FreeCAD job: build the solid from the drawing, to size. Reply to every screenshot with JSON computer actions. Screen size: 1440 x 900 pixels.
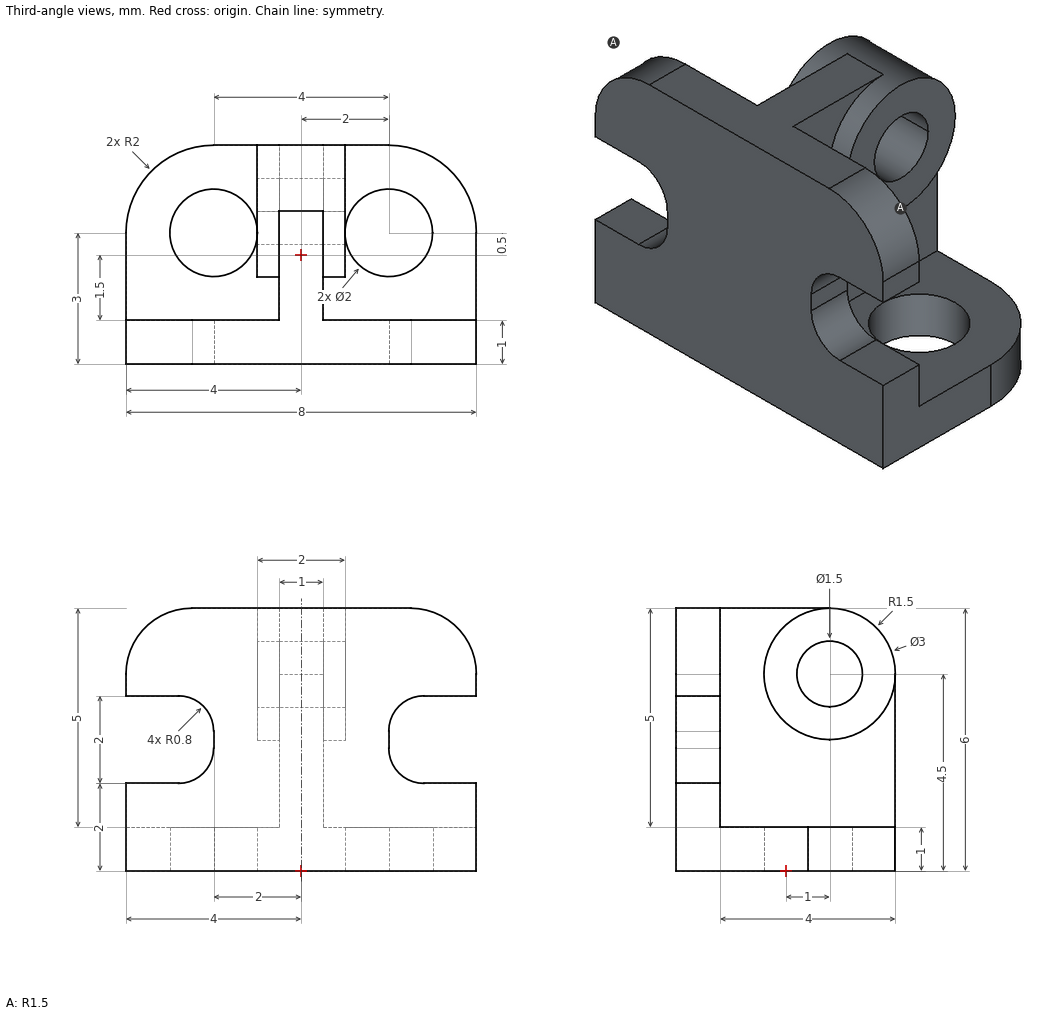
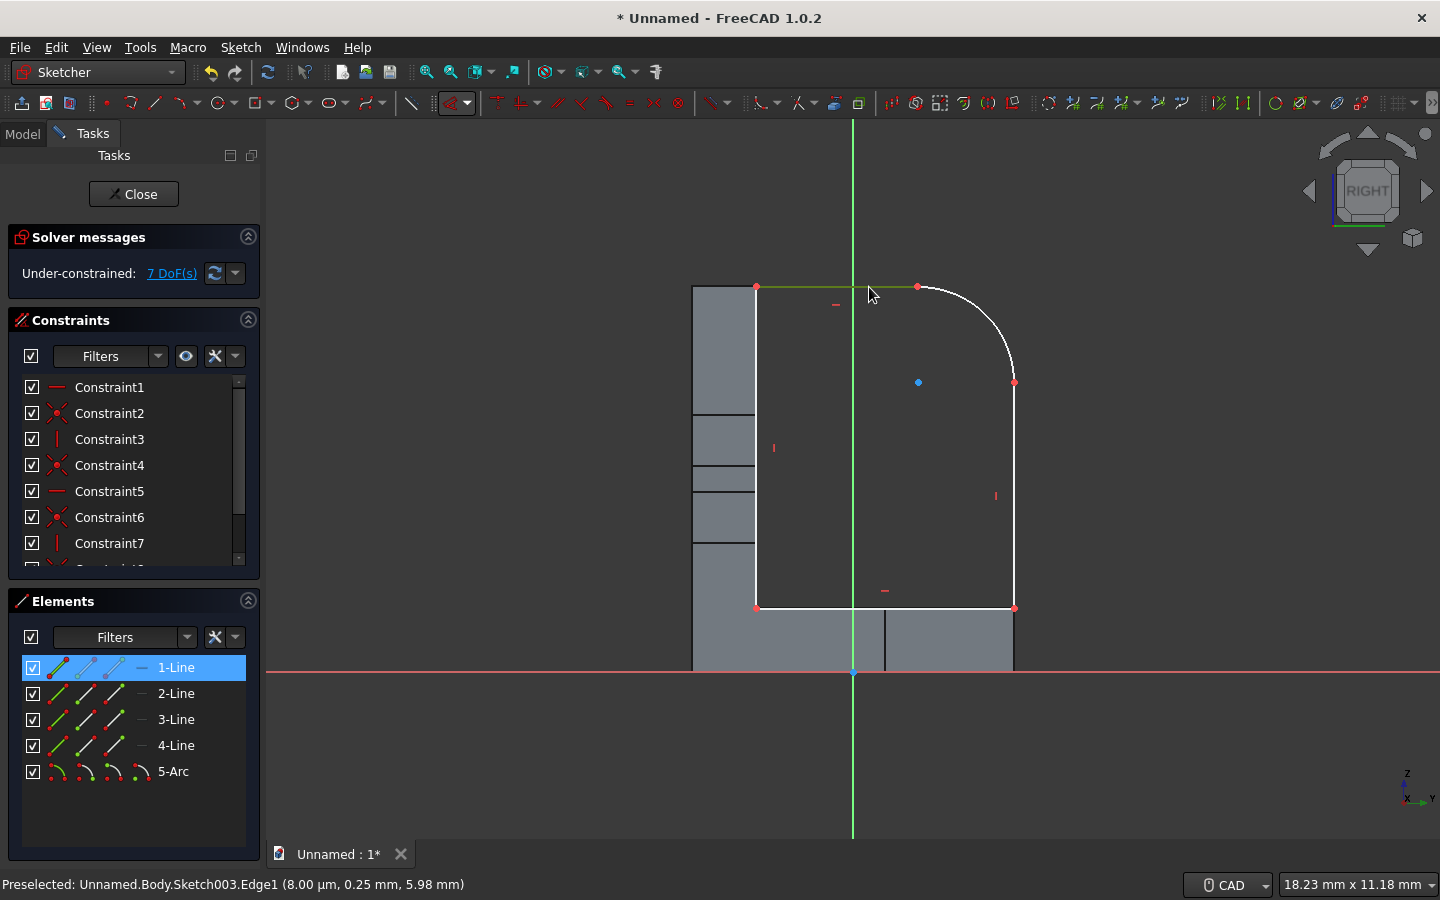
{"action": "left_click", "coordinate": [1004, 339]}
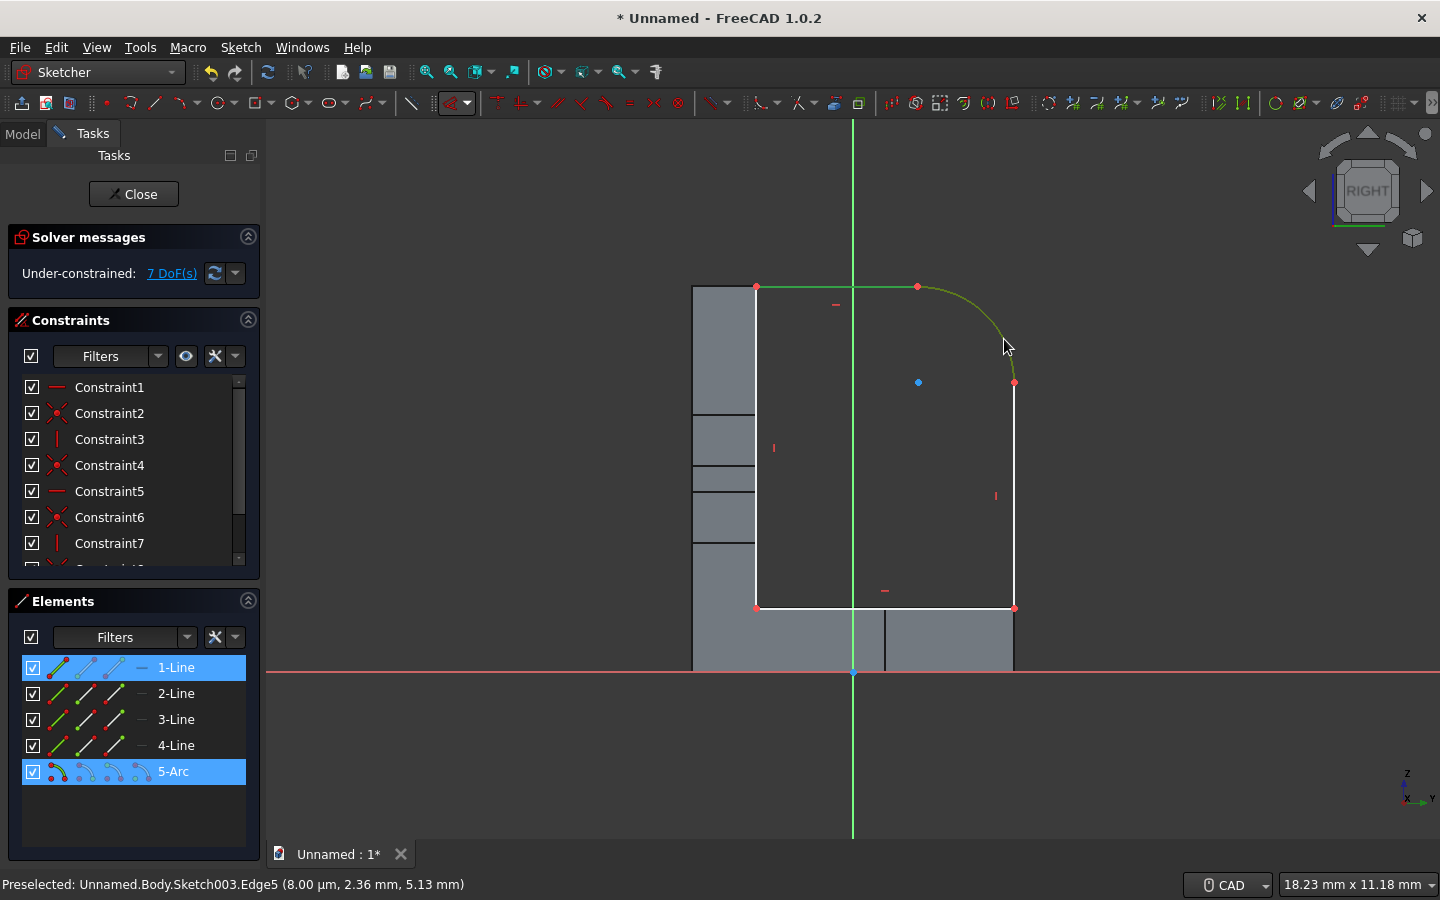
{"action": "left_click", "coordinate": [606, 104]}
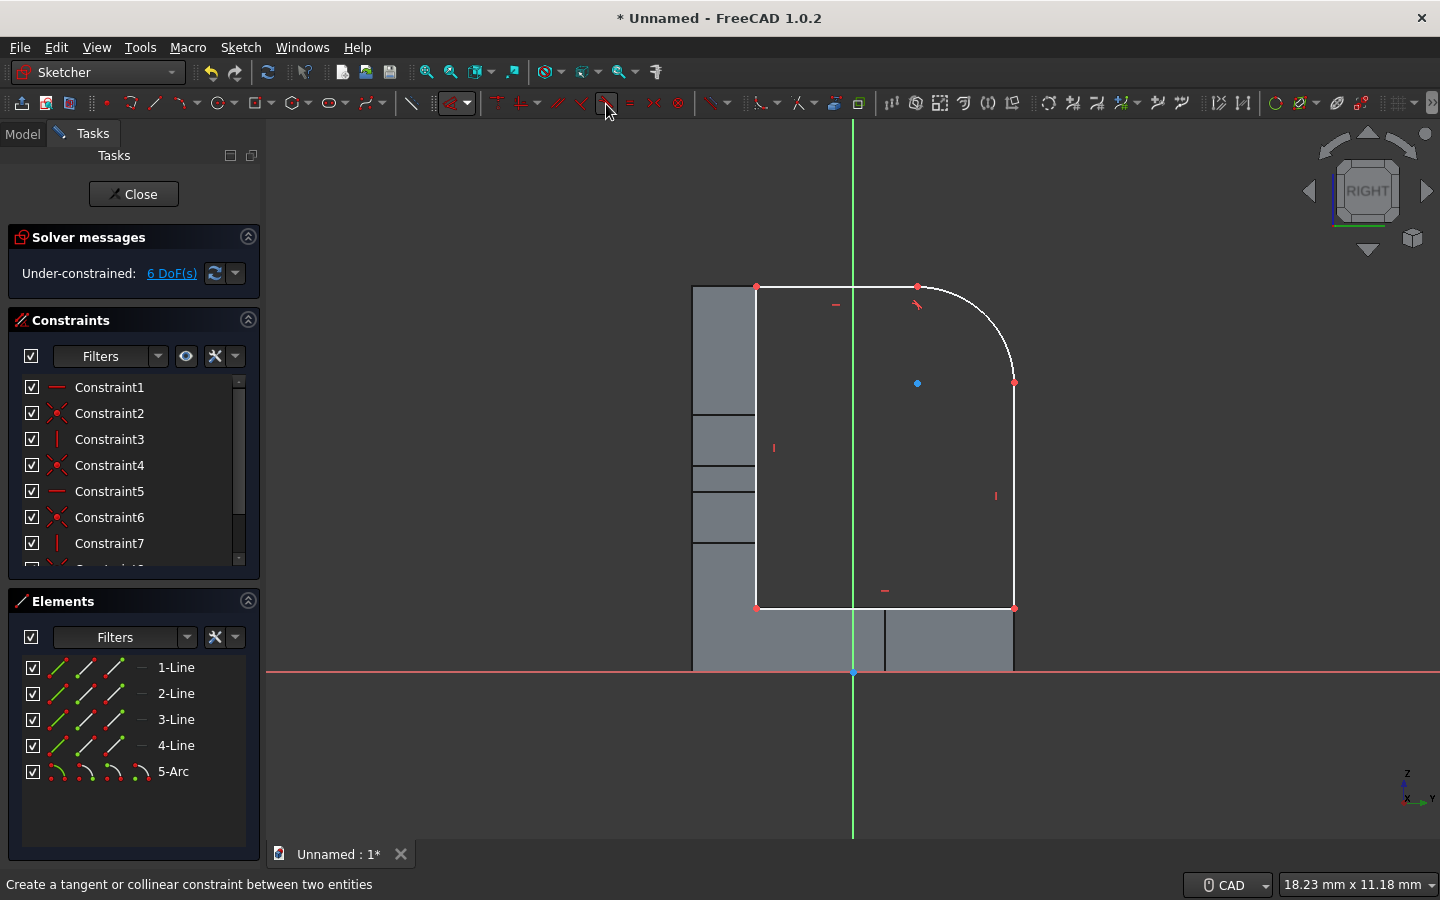
{"action": "left_click", "coordinate": [1014, 541]}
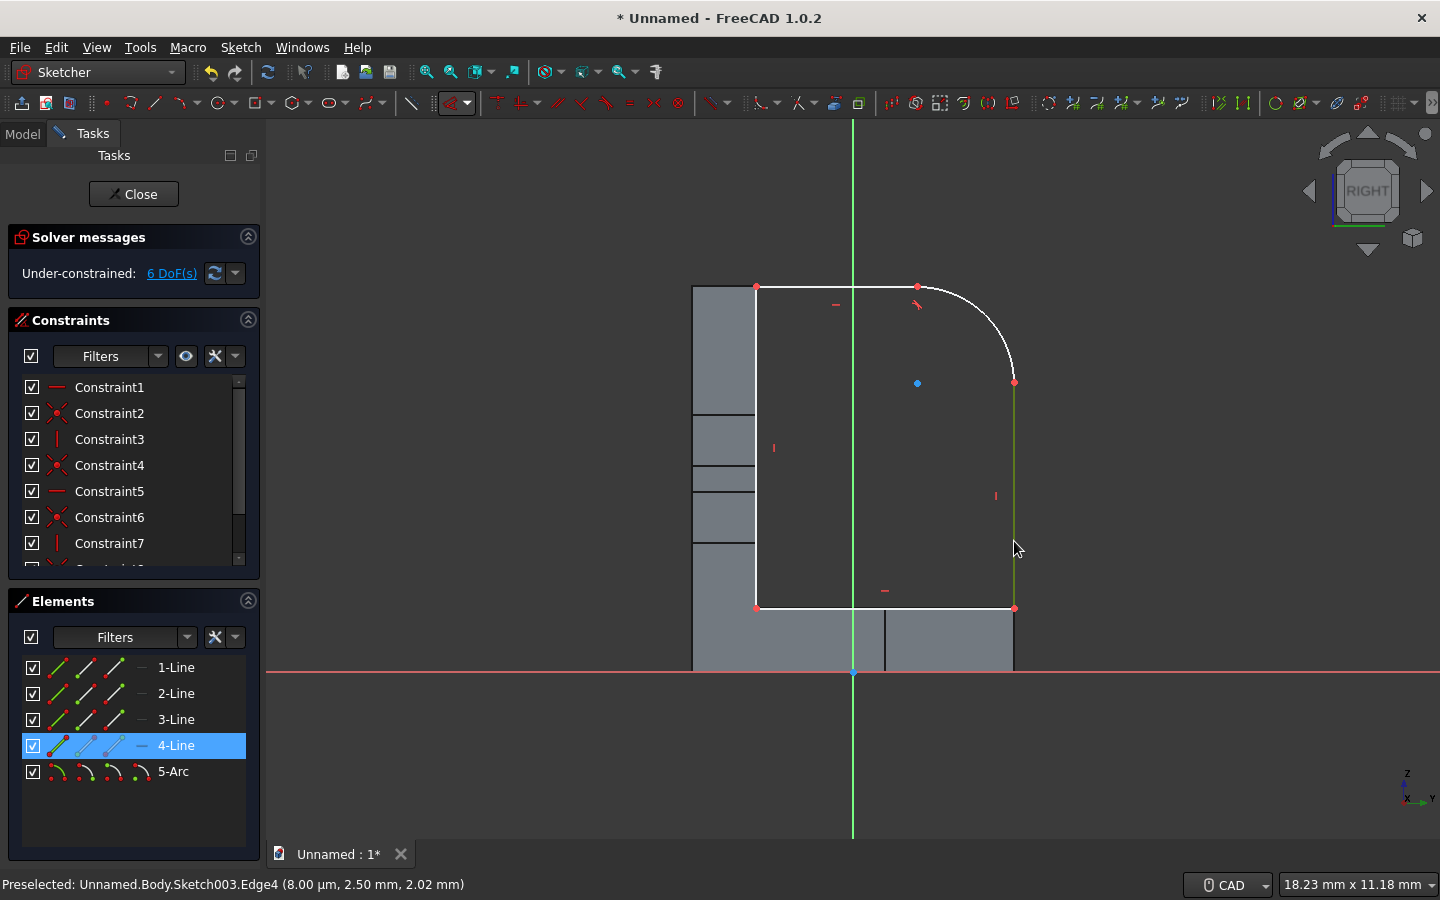
{"action": "left_click", "coordinate": [1003, 339]}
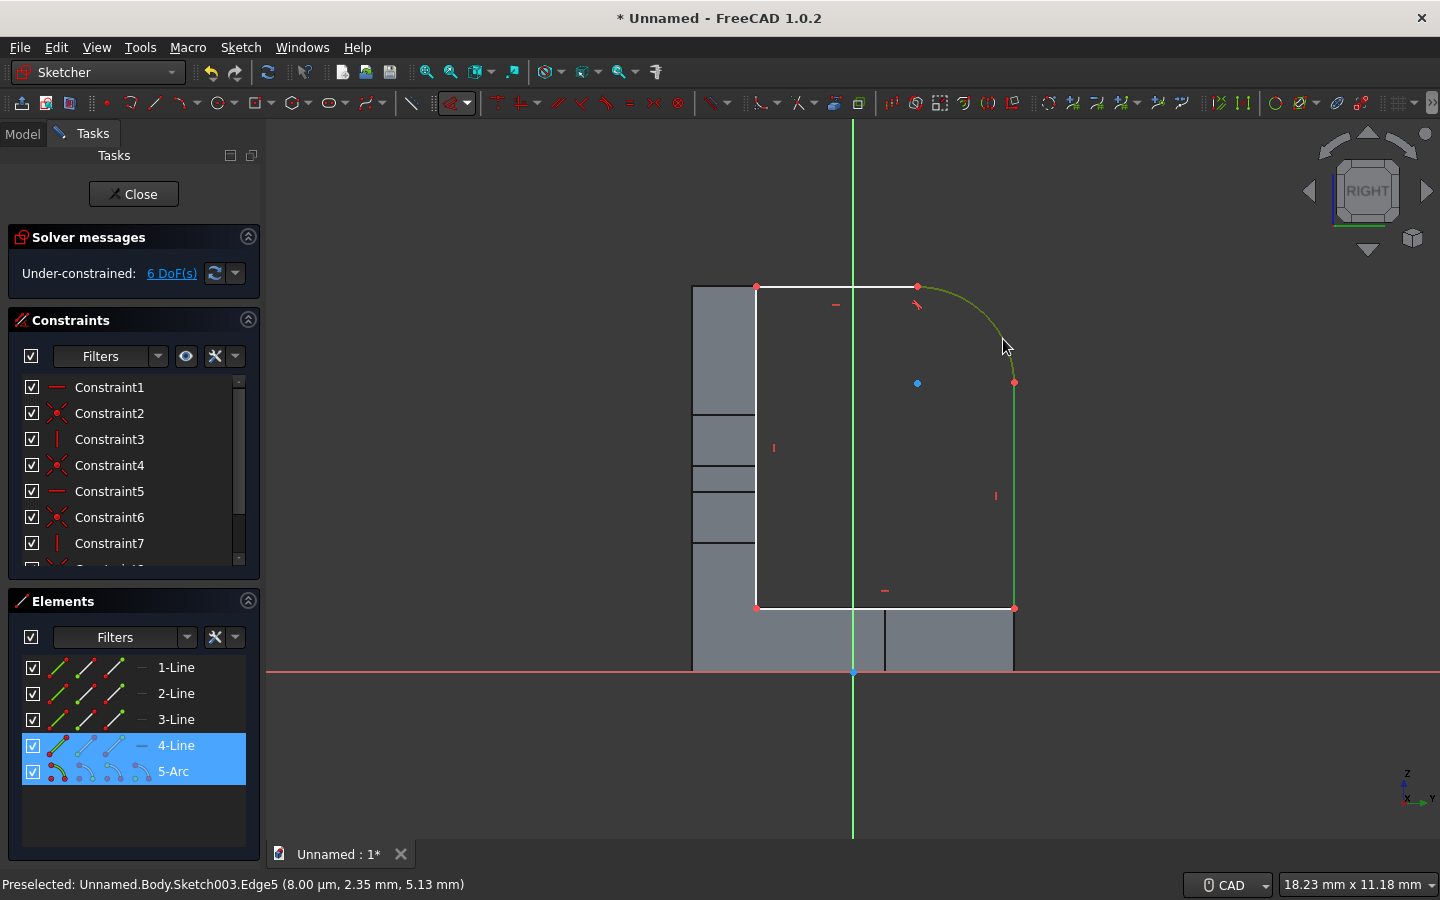
{"action": "left_click", "coordinate": [606, 104]}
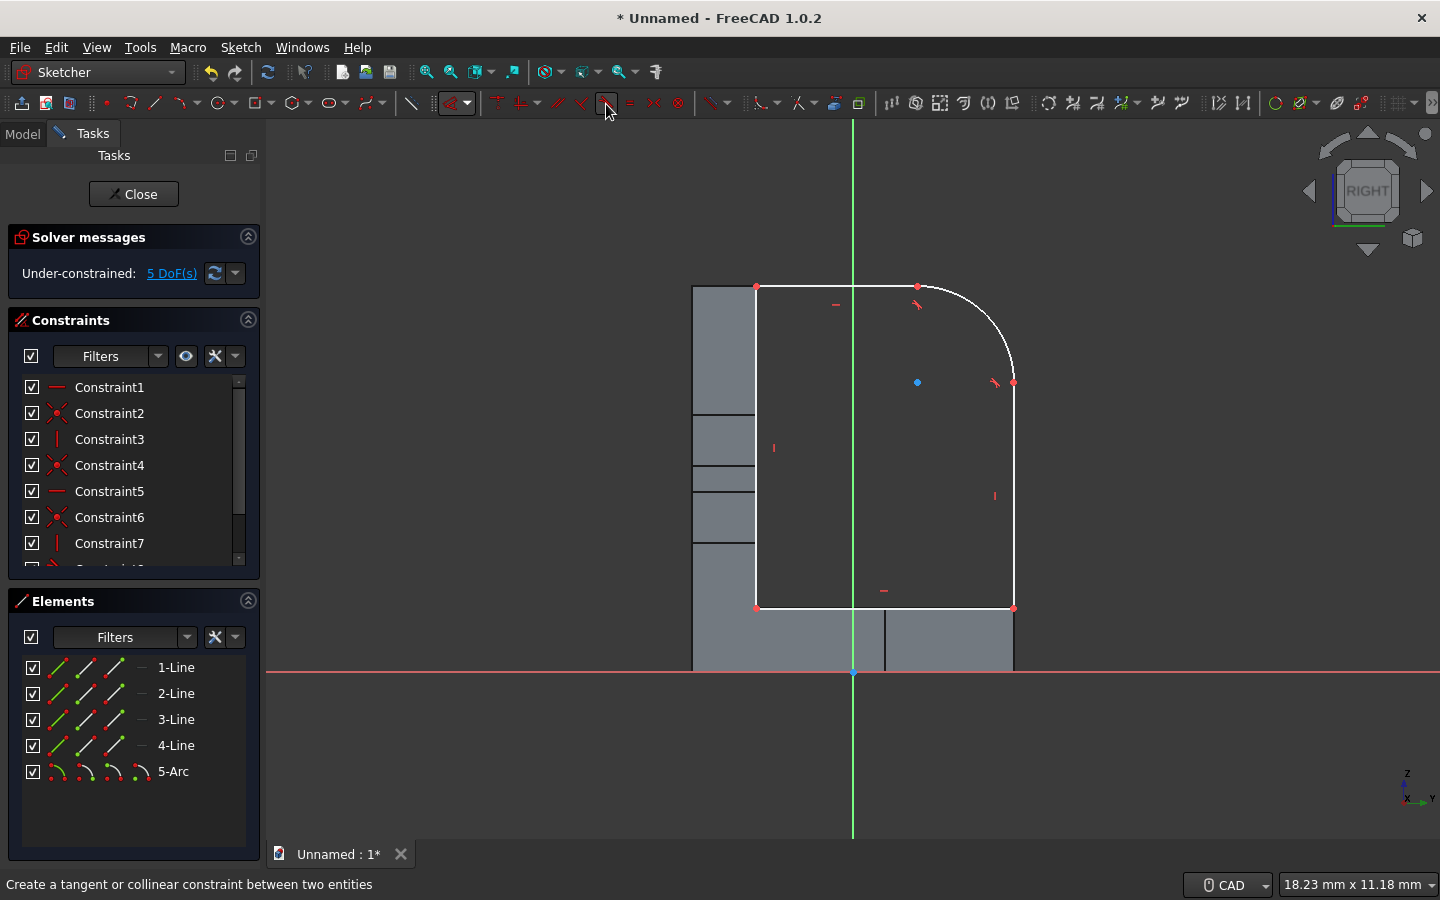
{"action": "left_click", "coordinate": [1003, 339]}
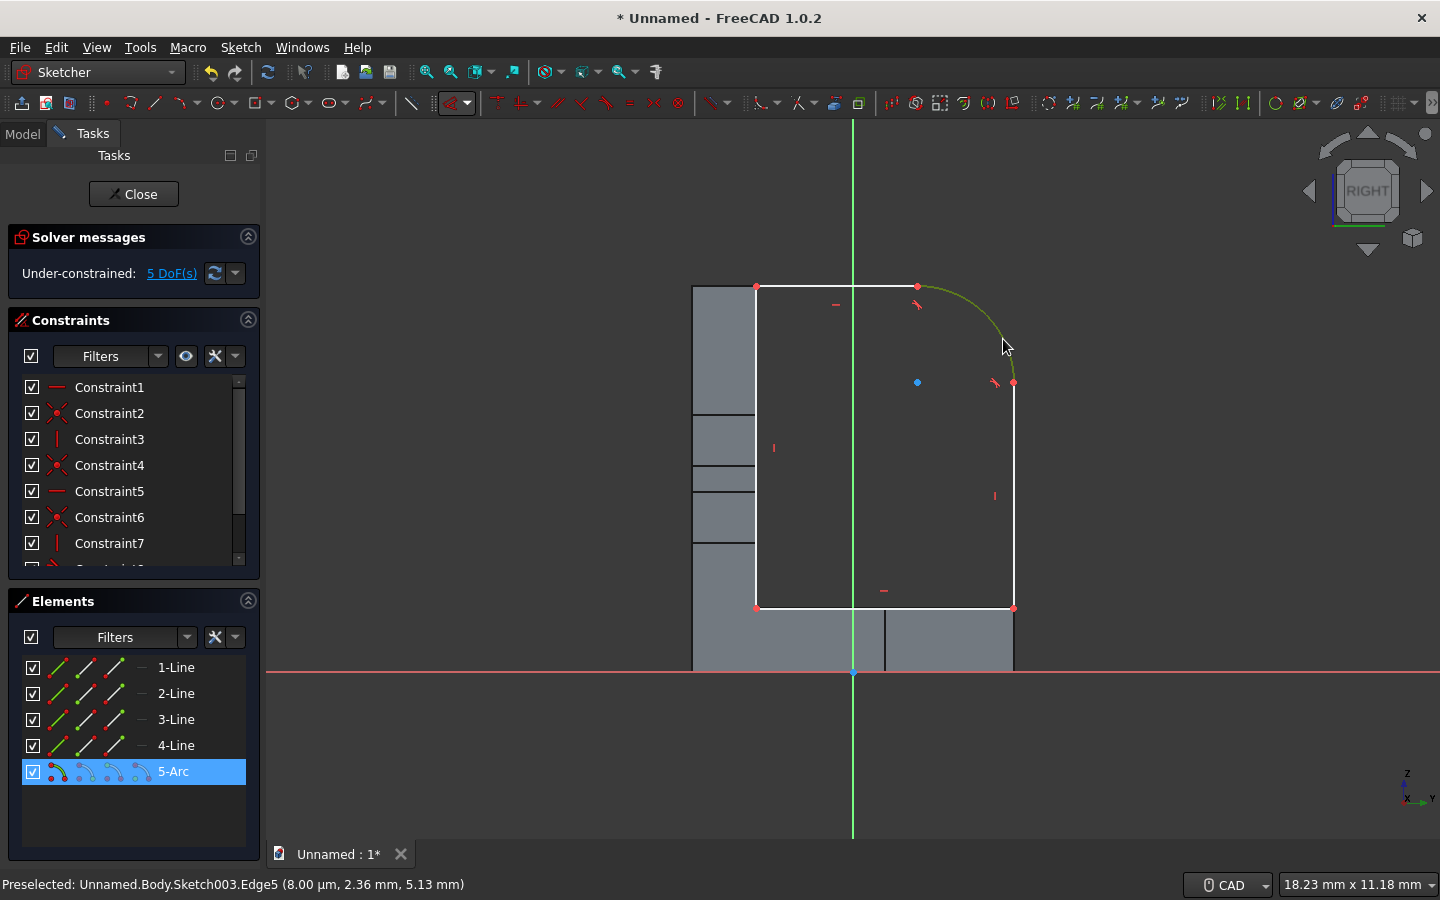
{"action": "left_click", "coordinate": [470, 104]}